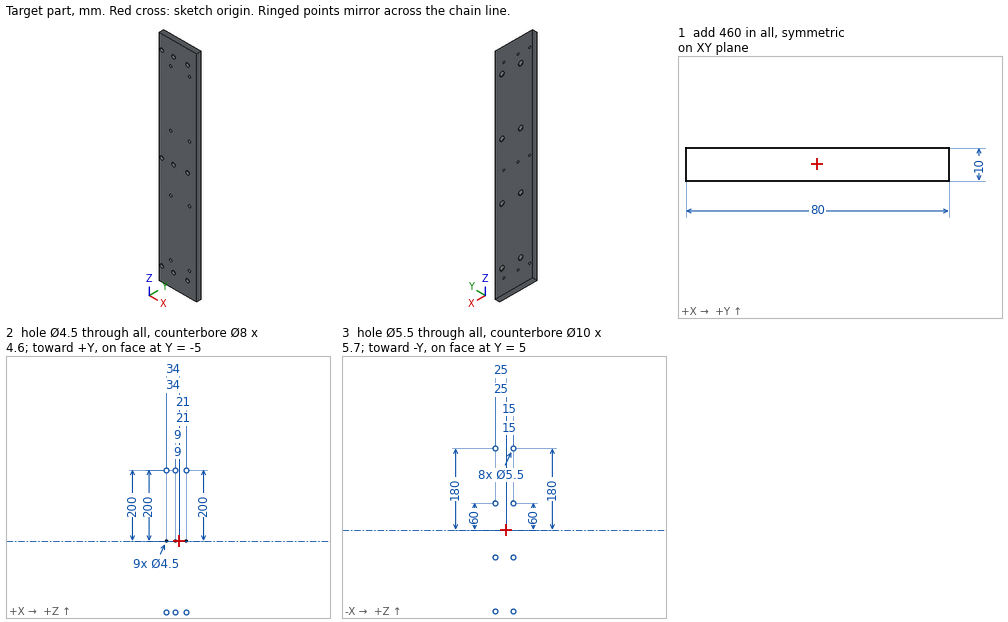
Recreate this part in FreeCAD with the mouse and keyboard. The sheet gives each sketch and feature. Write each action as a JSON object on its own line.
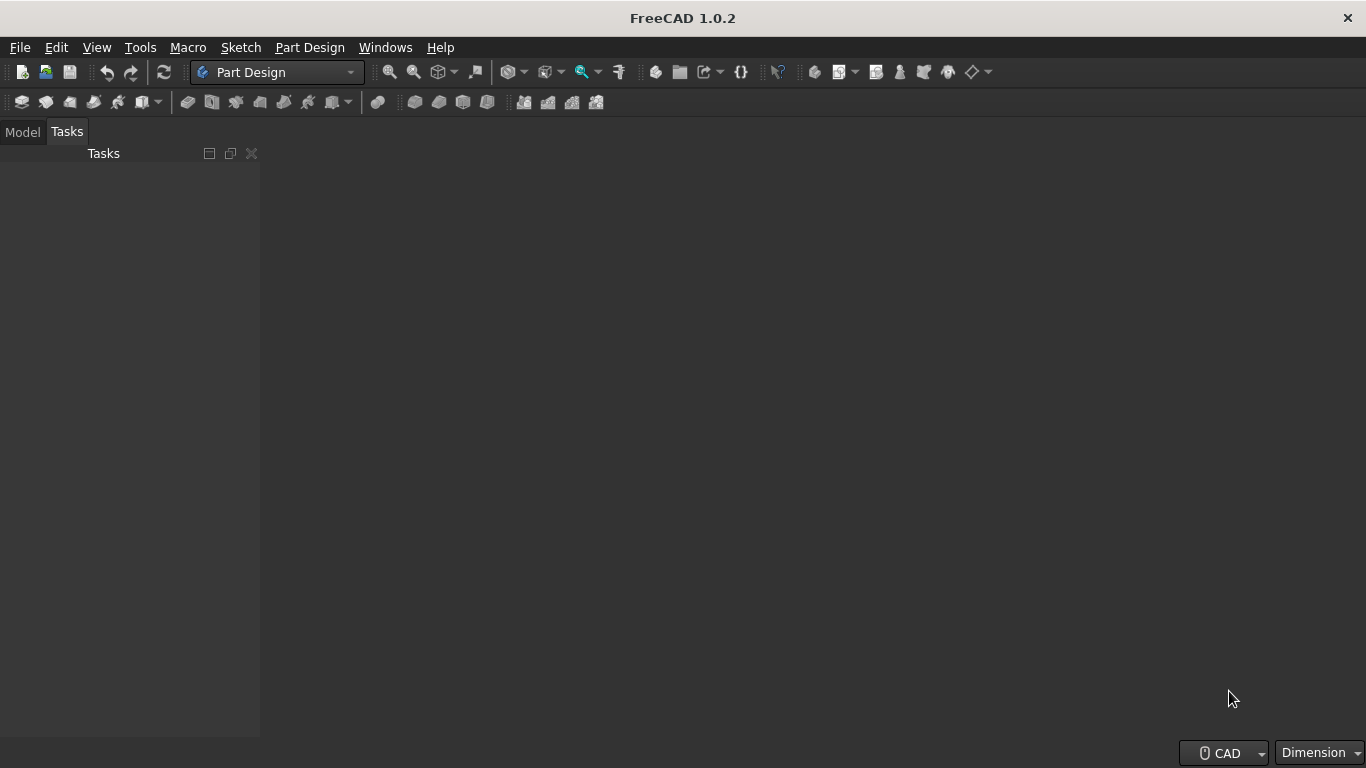
{"action": "key", "text": "ctrl+n"}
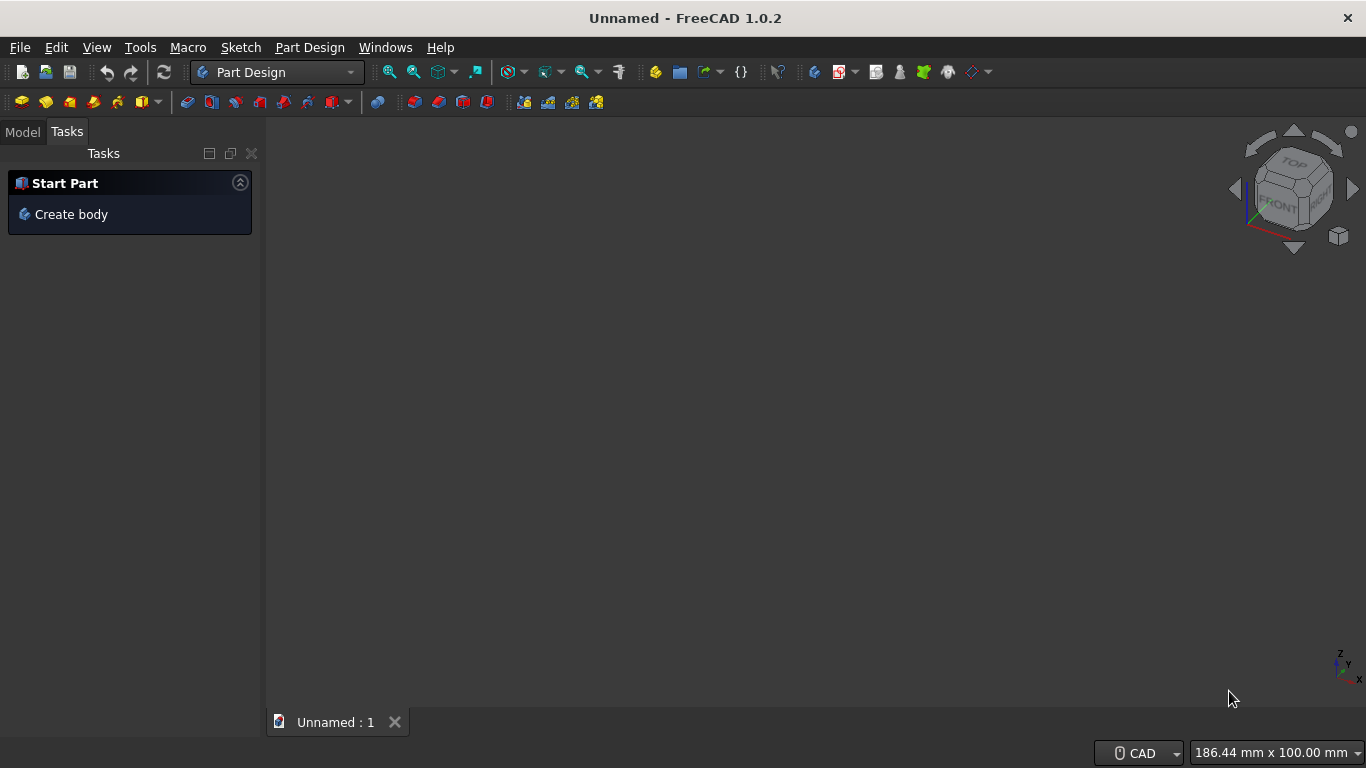
{"action": "left_click", "coordinate": [840, 72]}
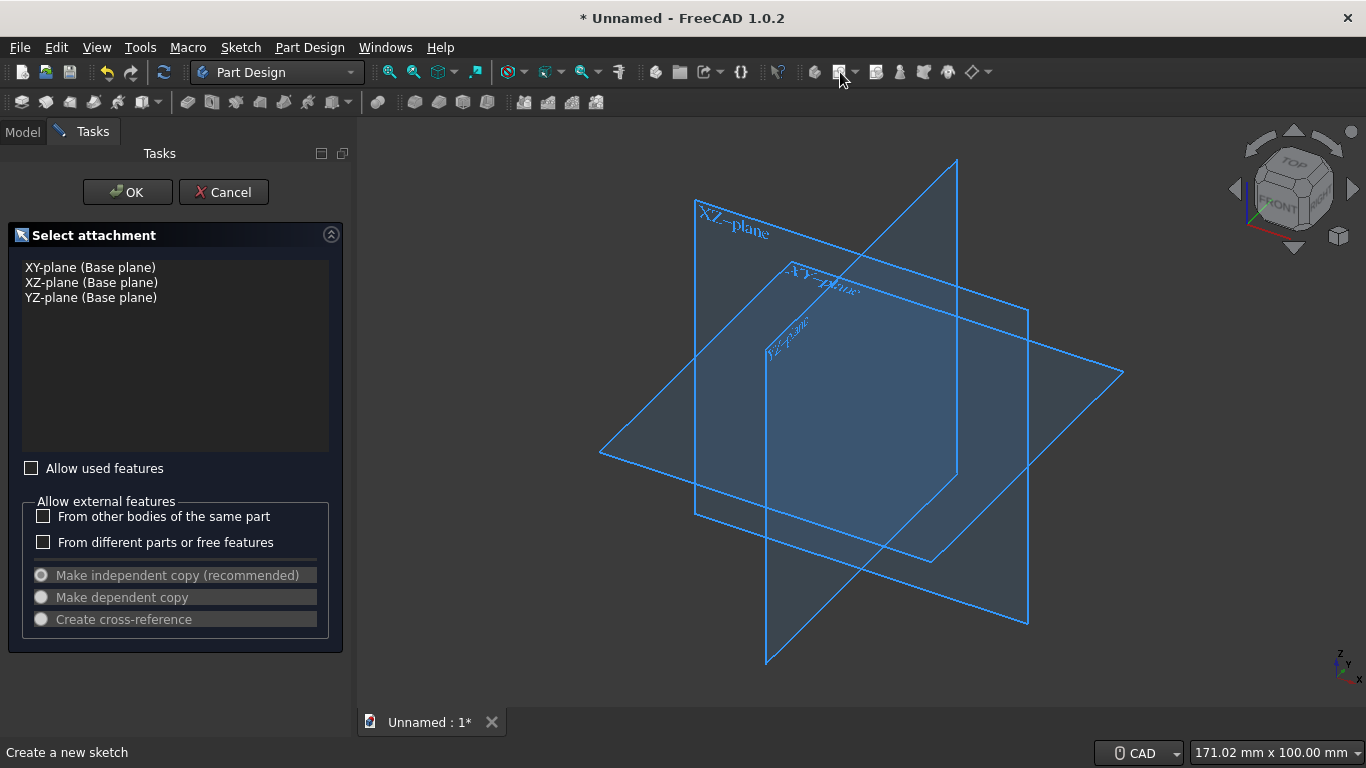
{"action": "left_click", "coordinate": [82, 268]}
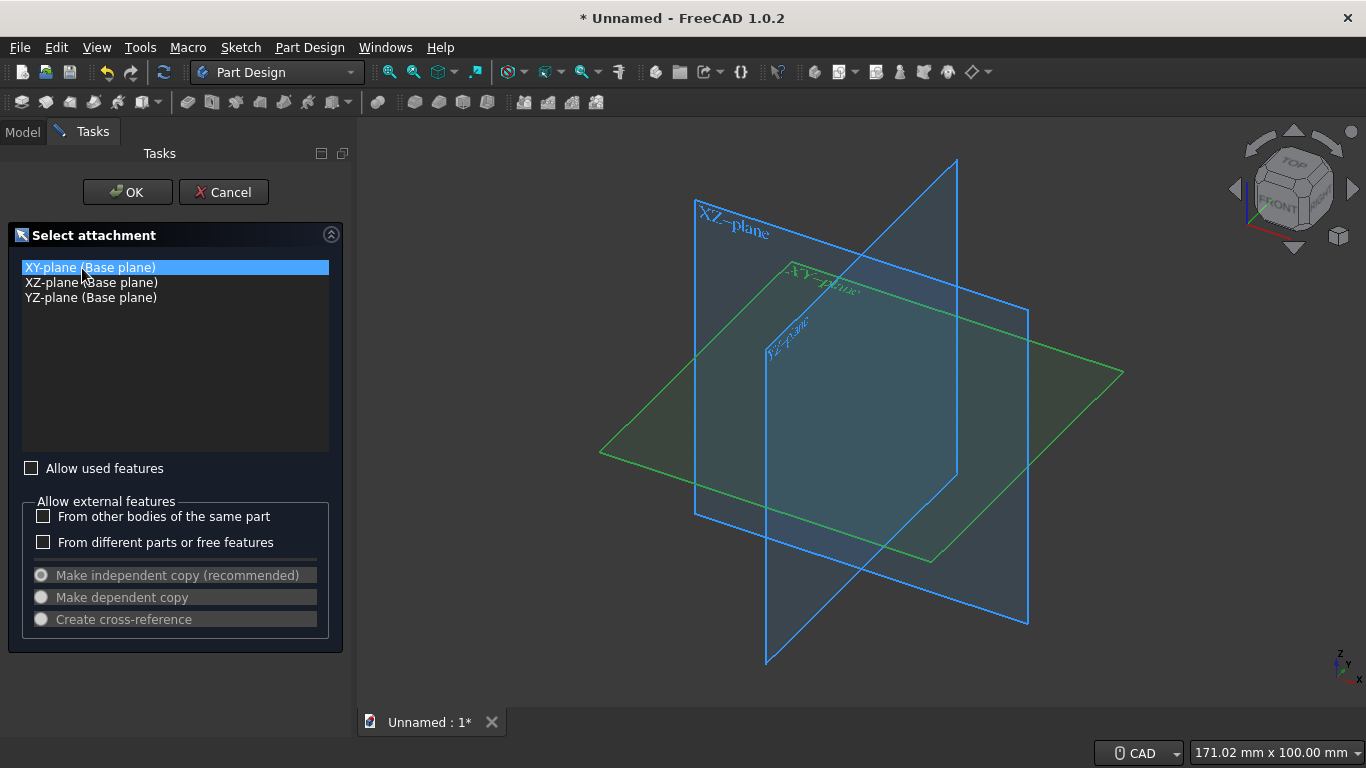
{"action": "left_click", "coordinate": [128, 192]}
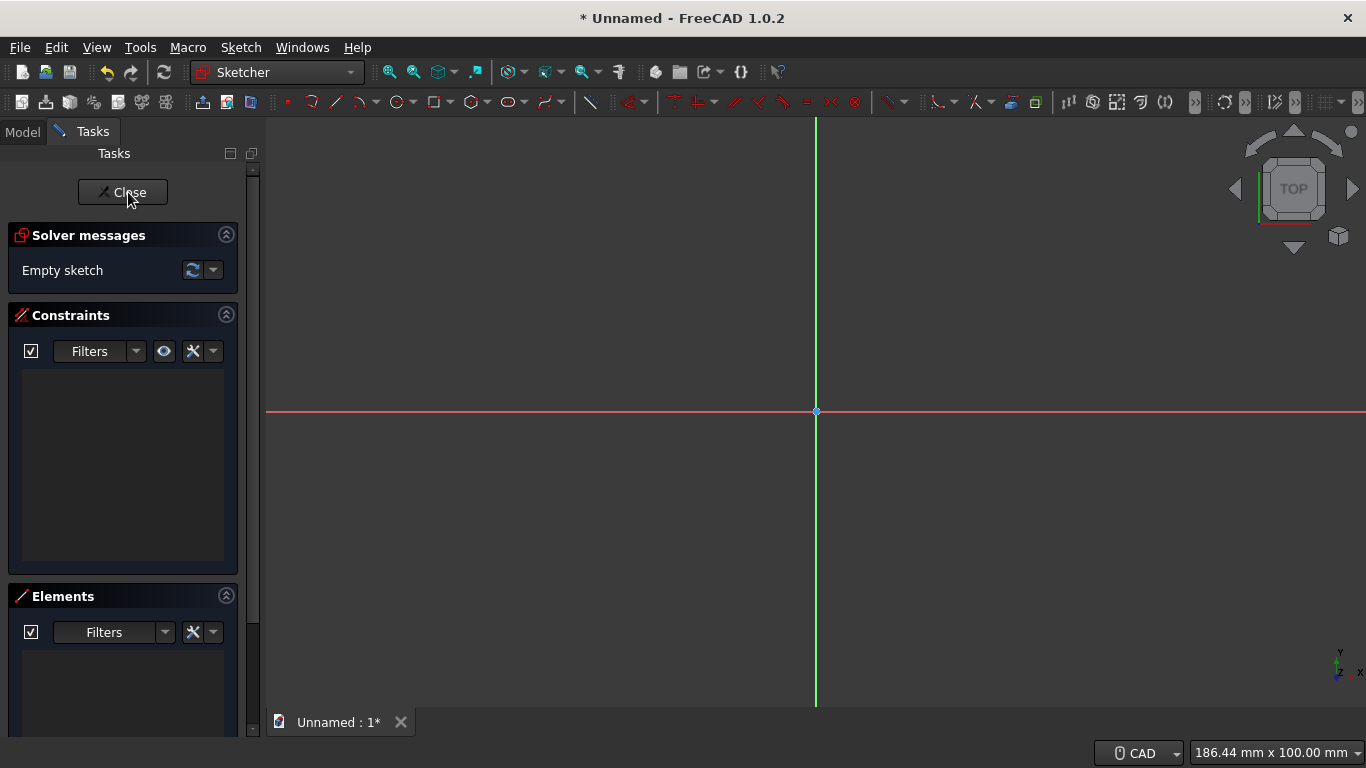
{"action": "scroll", "coordinate": [955, 412], "scroll_direction": "up", "scroll_amount": 2}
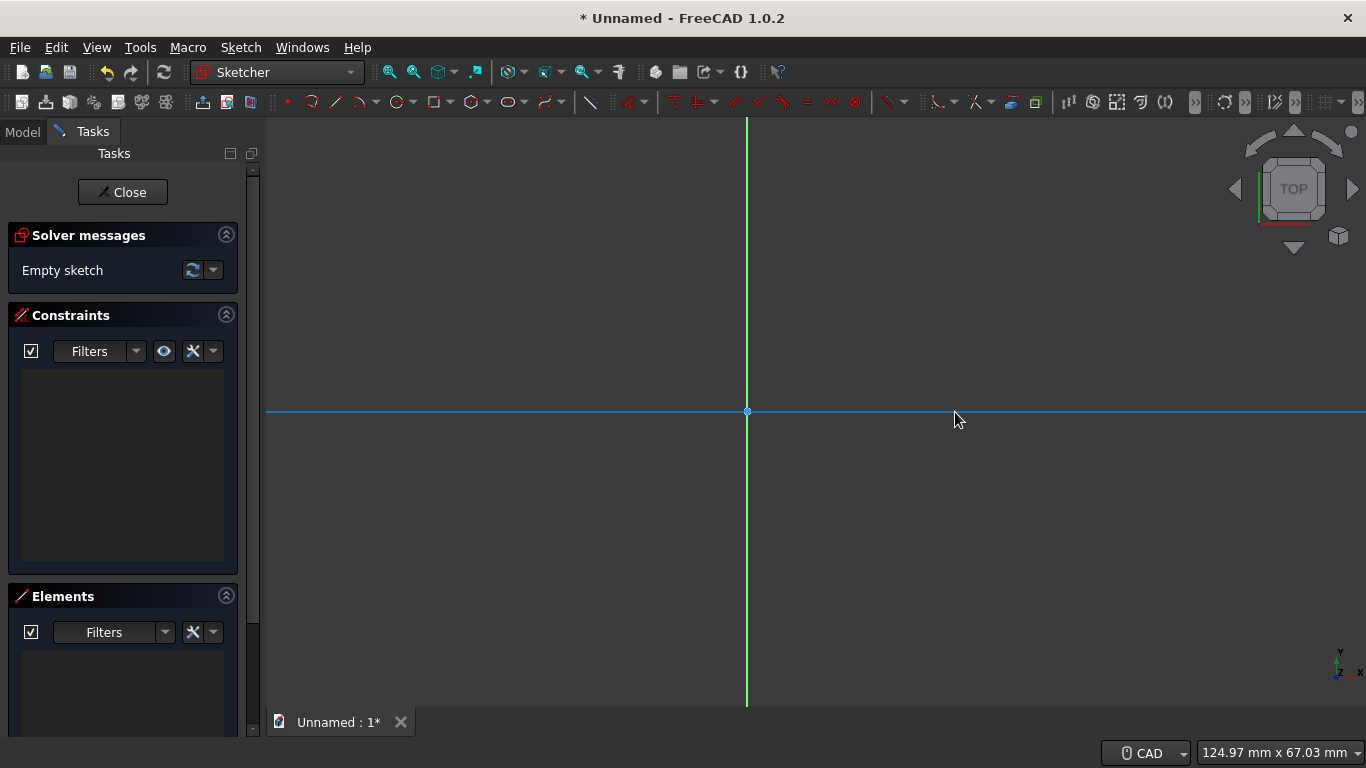
{"action": "key", "text": "g v"}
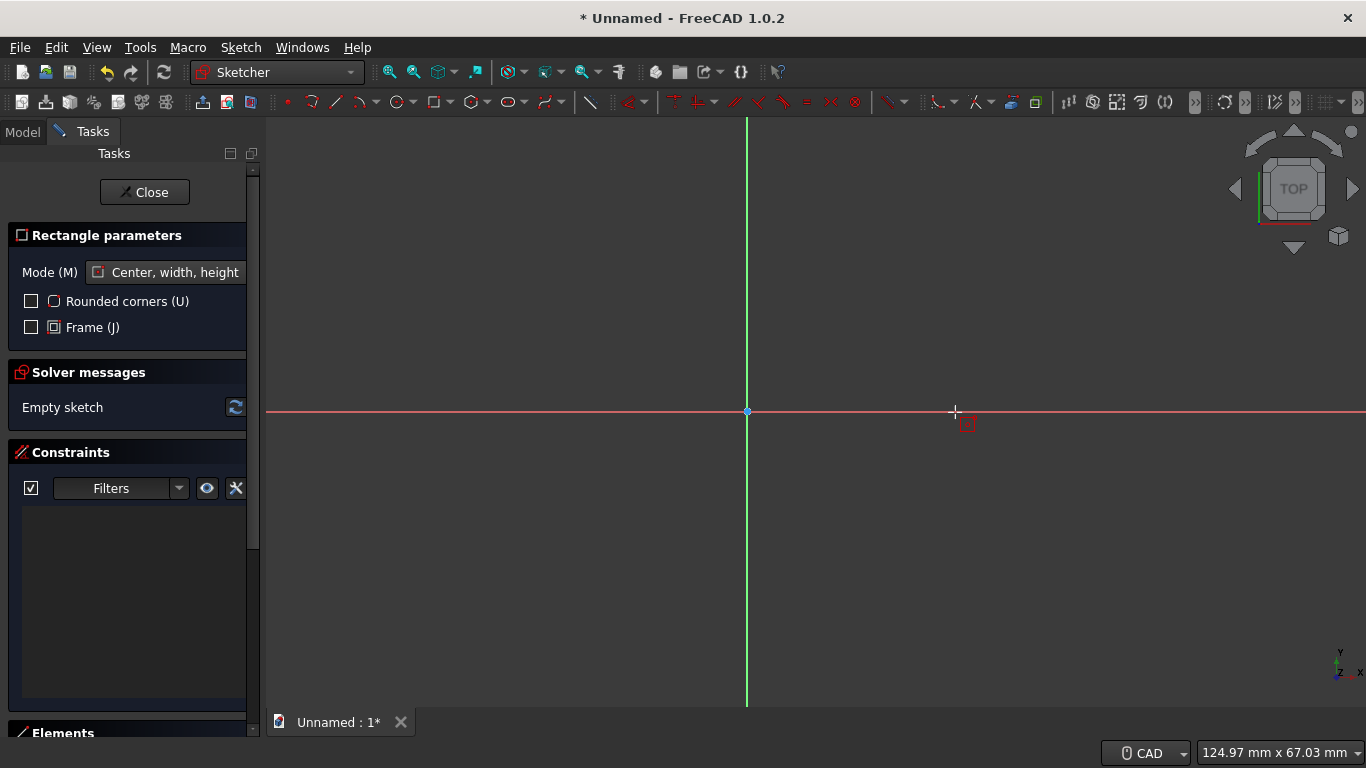
{"action": "left_click", "coordinate": [747, 412]}
{"action": "mouse_move", "coordinate": [1099, 368]}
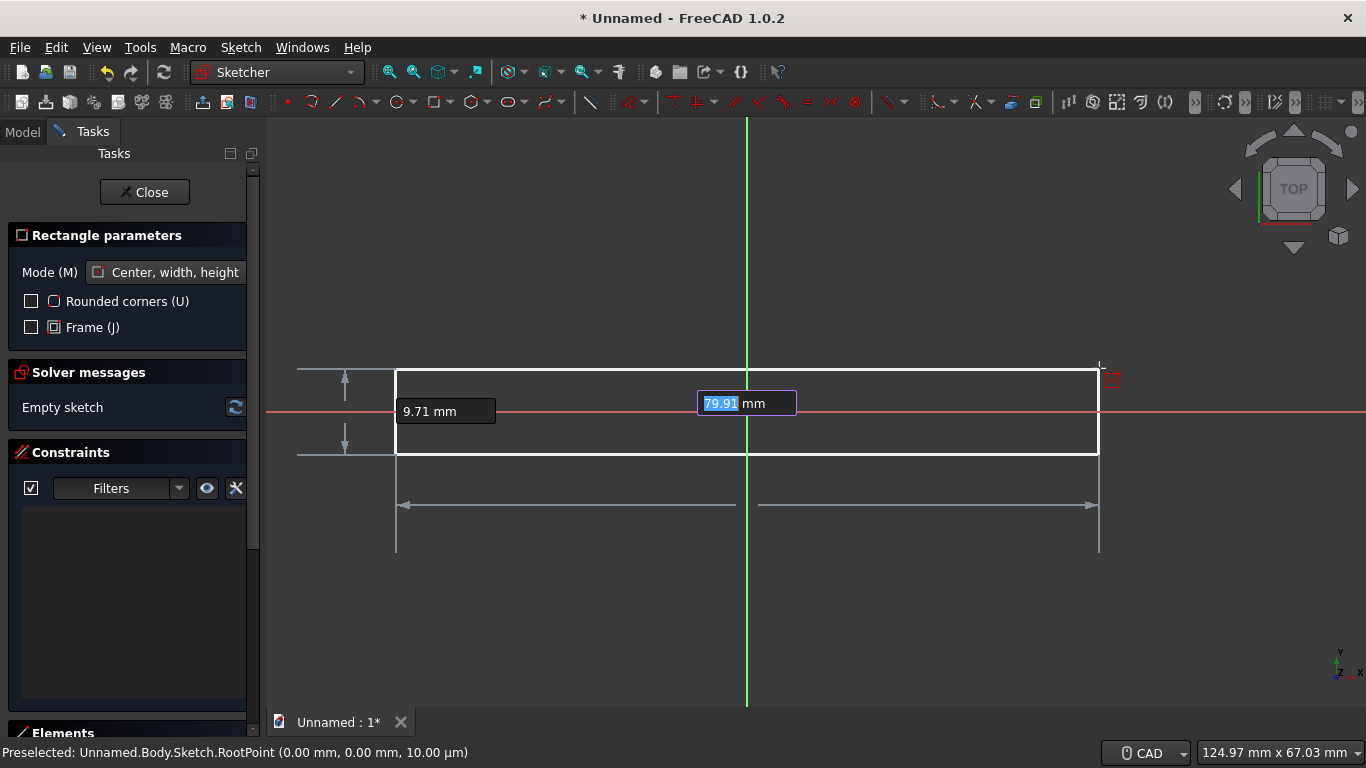
{"action": "type", "text": "80"}
{"action": "key", "text": "Tab"}
{"action": "type", "text": "10"}
{"action": "key", "text": "Return"}
{"action": "key", "text": "Escape"}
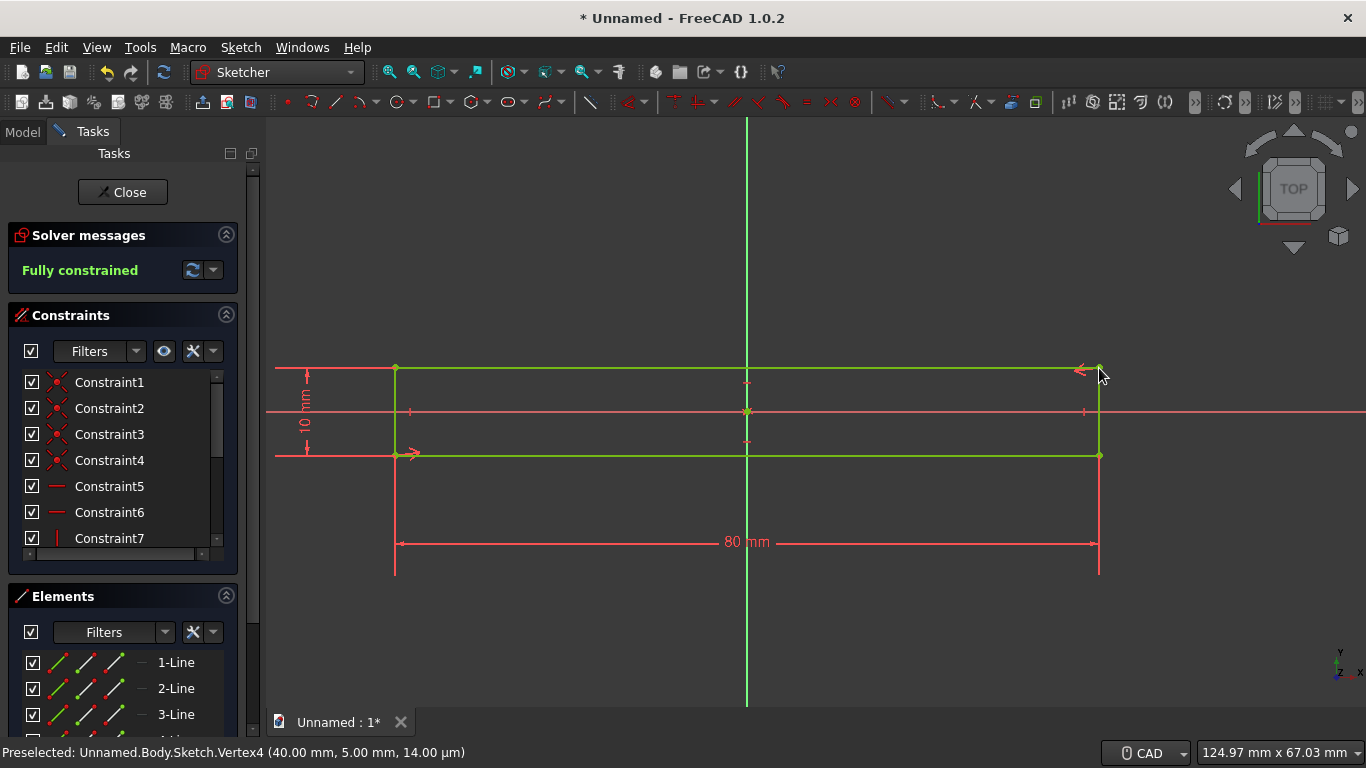
{"action": "left_click", "coordinate": [123, 192]}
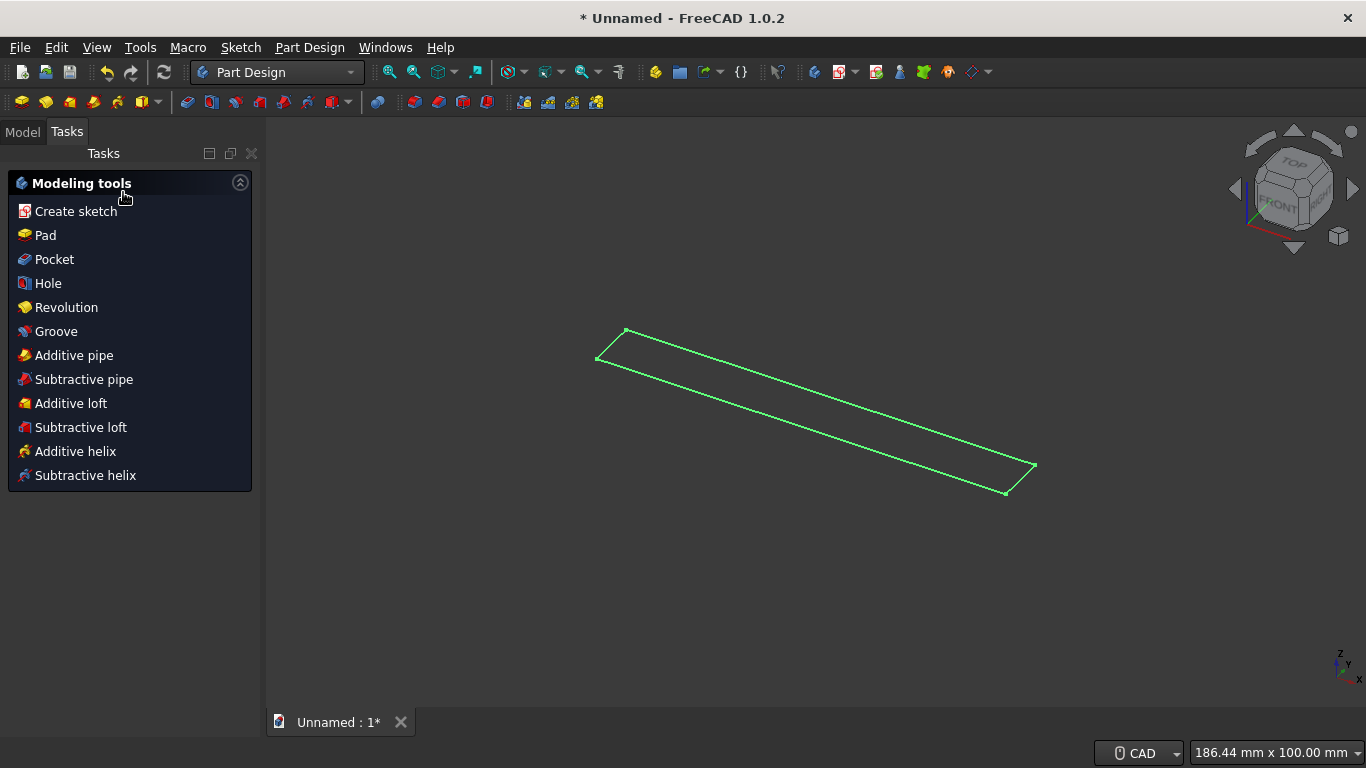
{"action": "left_click", "coordinate": [22, 102]}